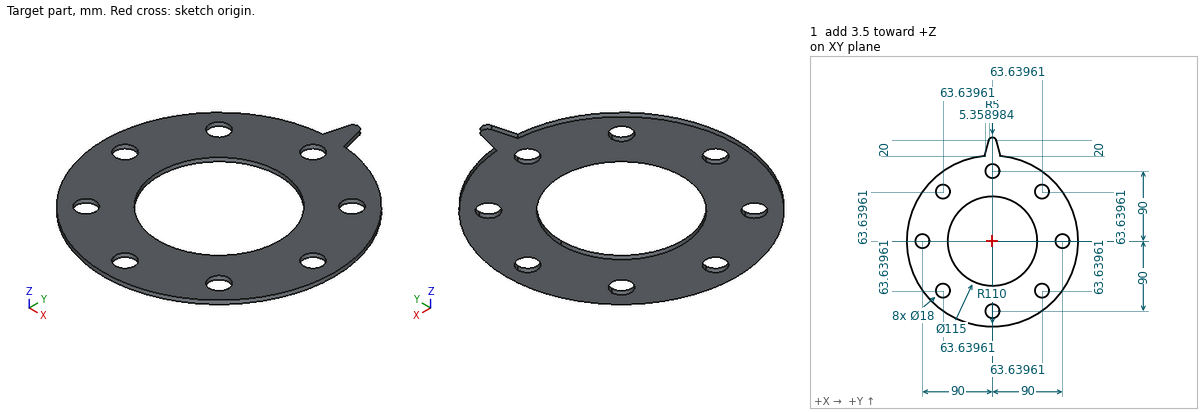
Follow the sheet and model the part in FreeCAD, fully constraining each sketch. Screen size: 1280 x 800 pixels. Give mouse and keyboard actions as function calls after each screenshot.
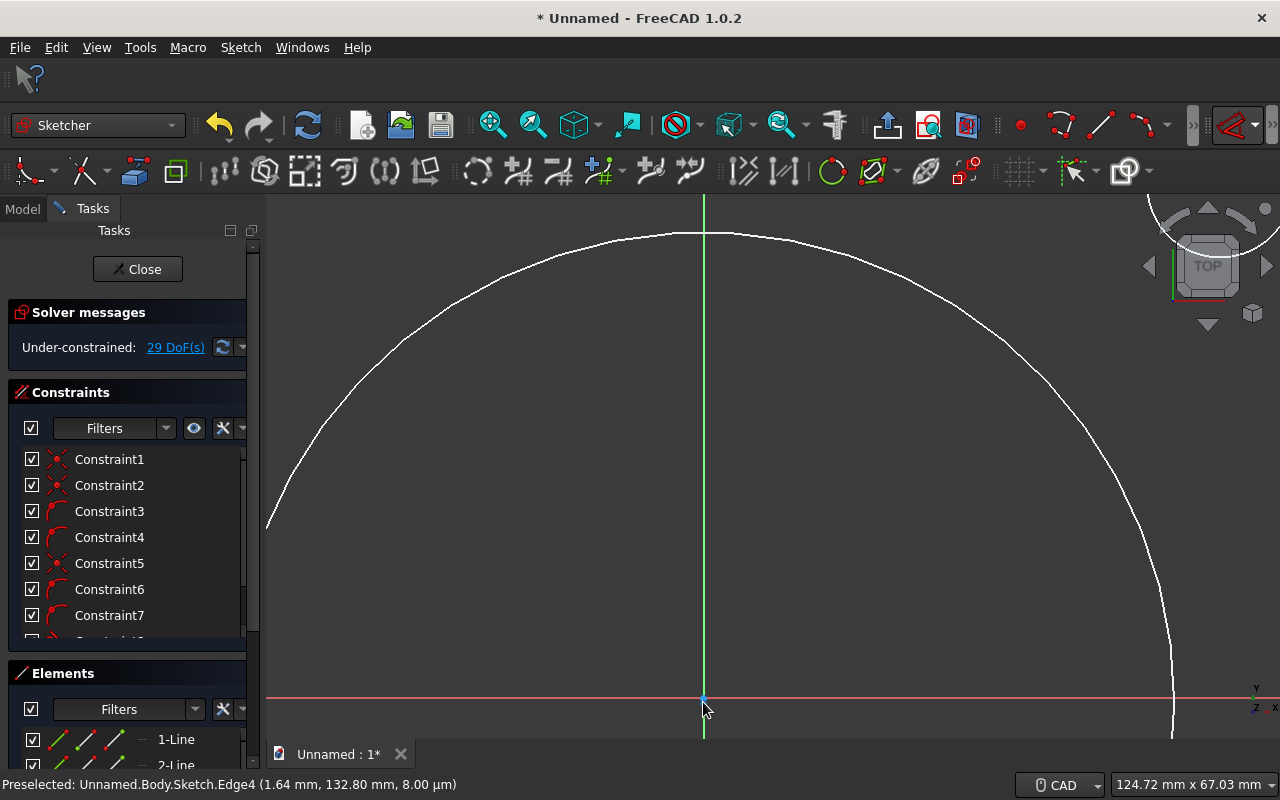
drag(693, 688, 714, 713)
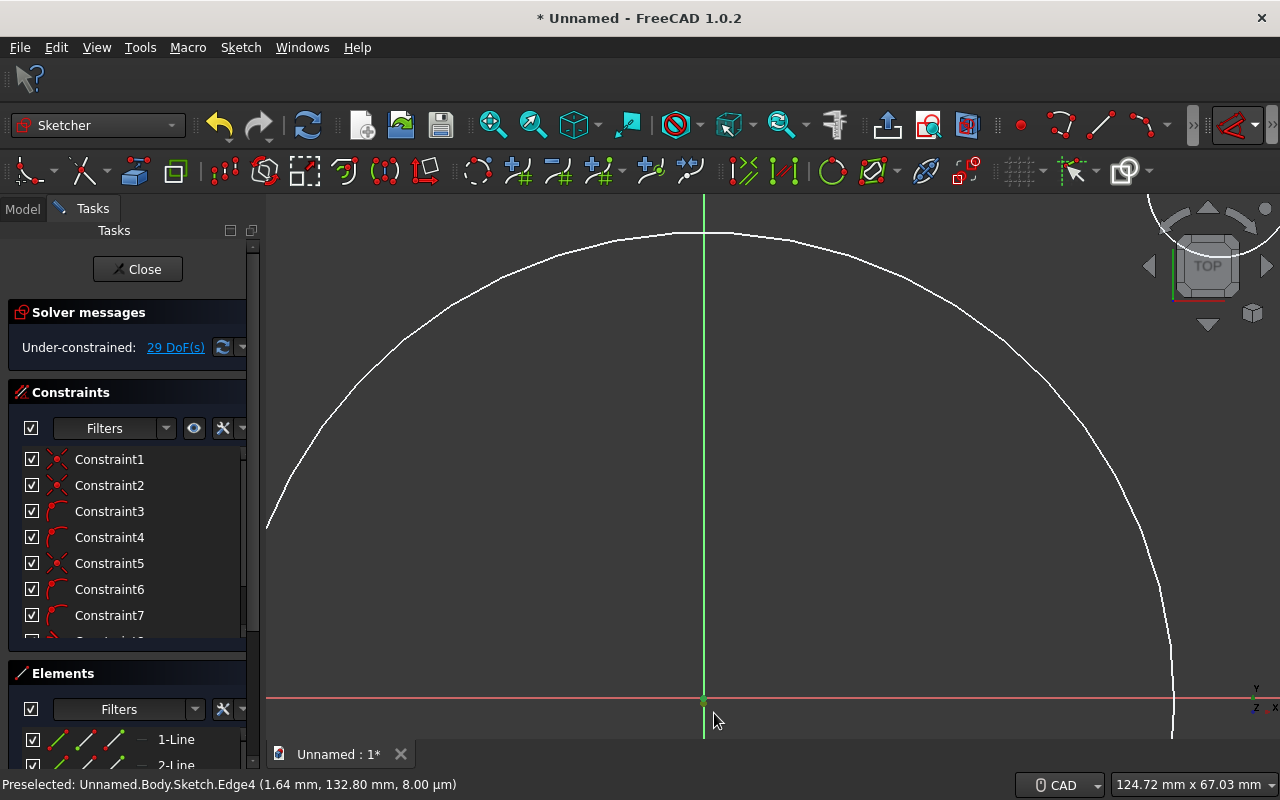
key(c)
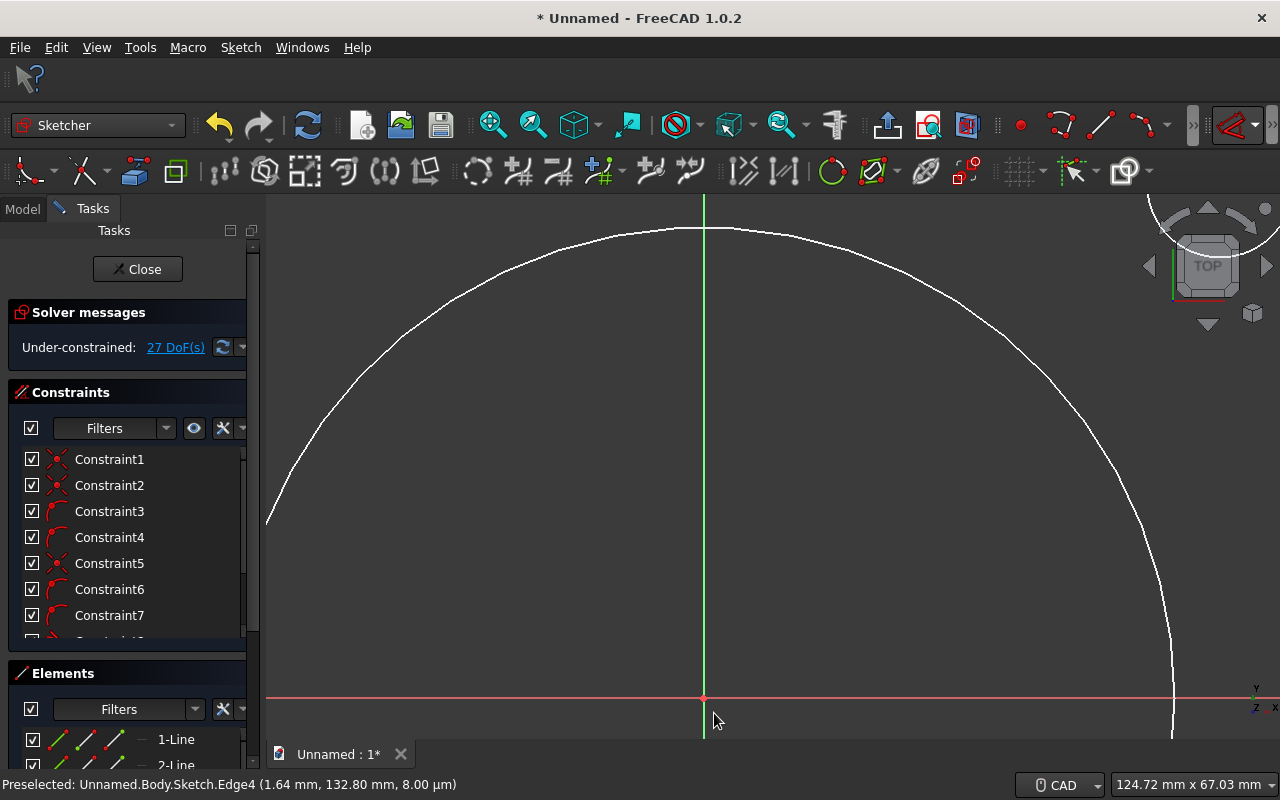
scroll(705, 439, down, 9)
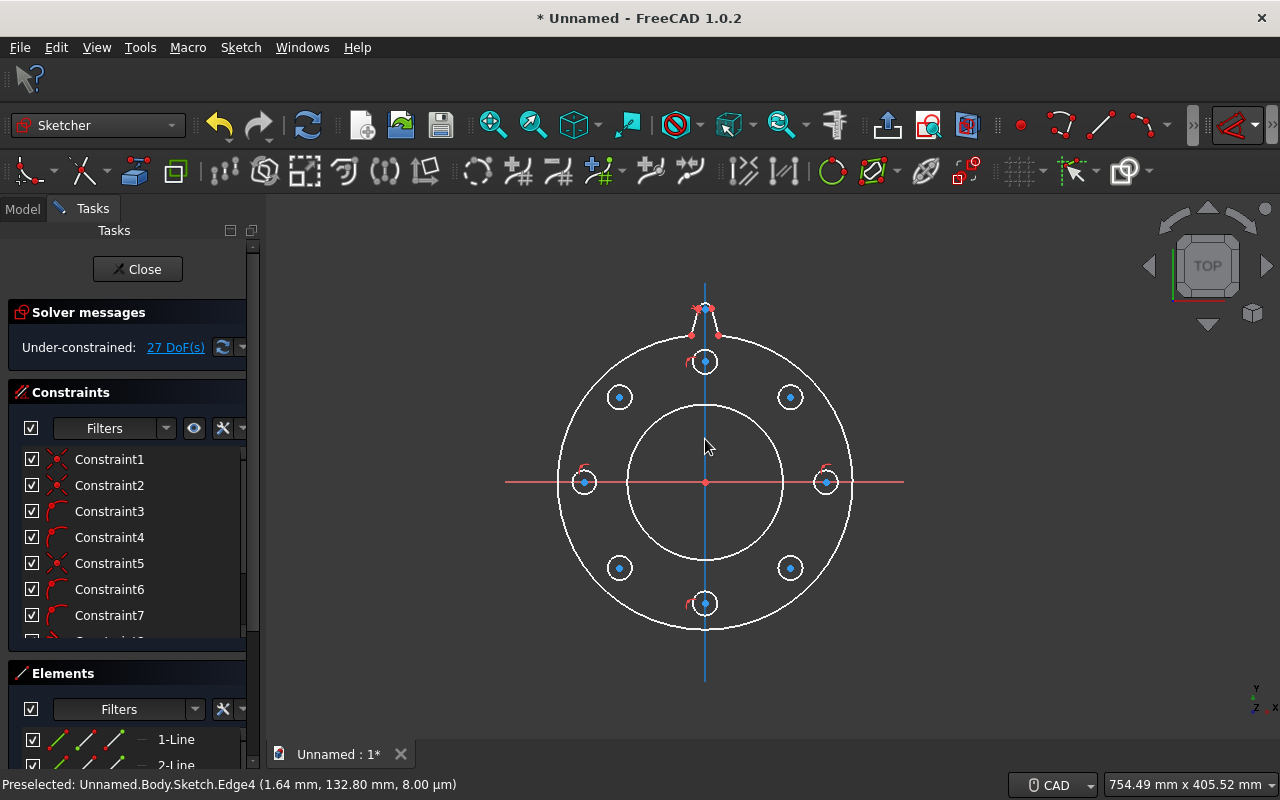
click(628, 559)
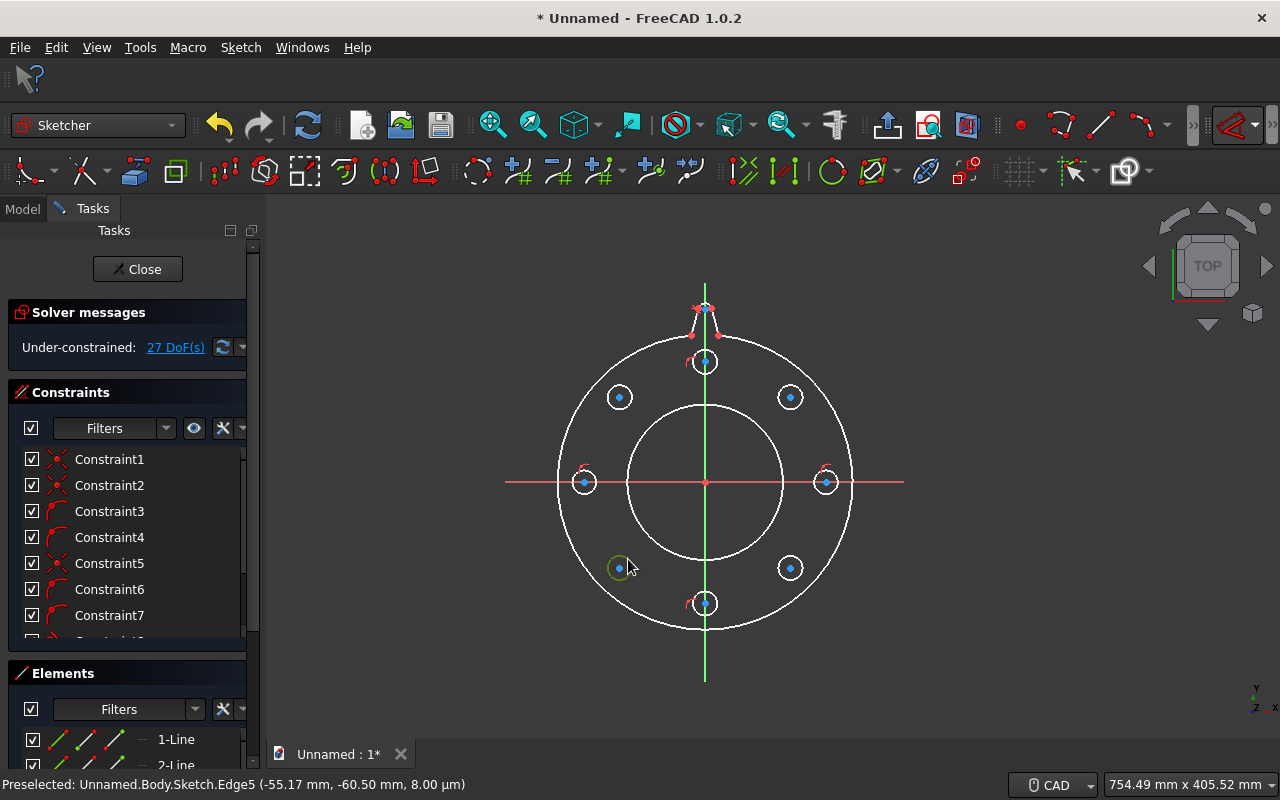
click(705, 591)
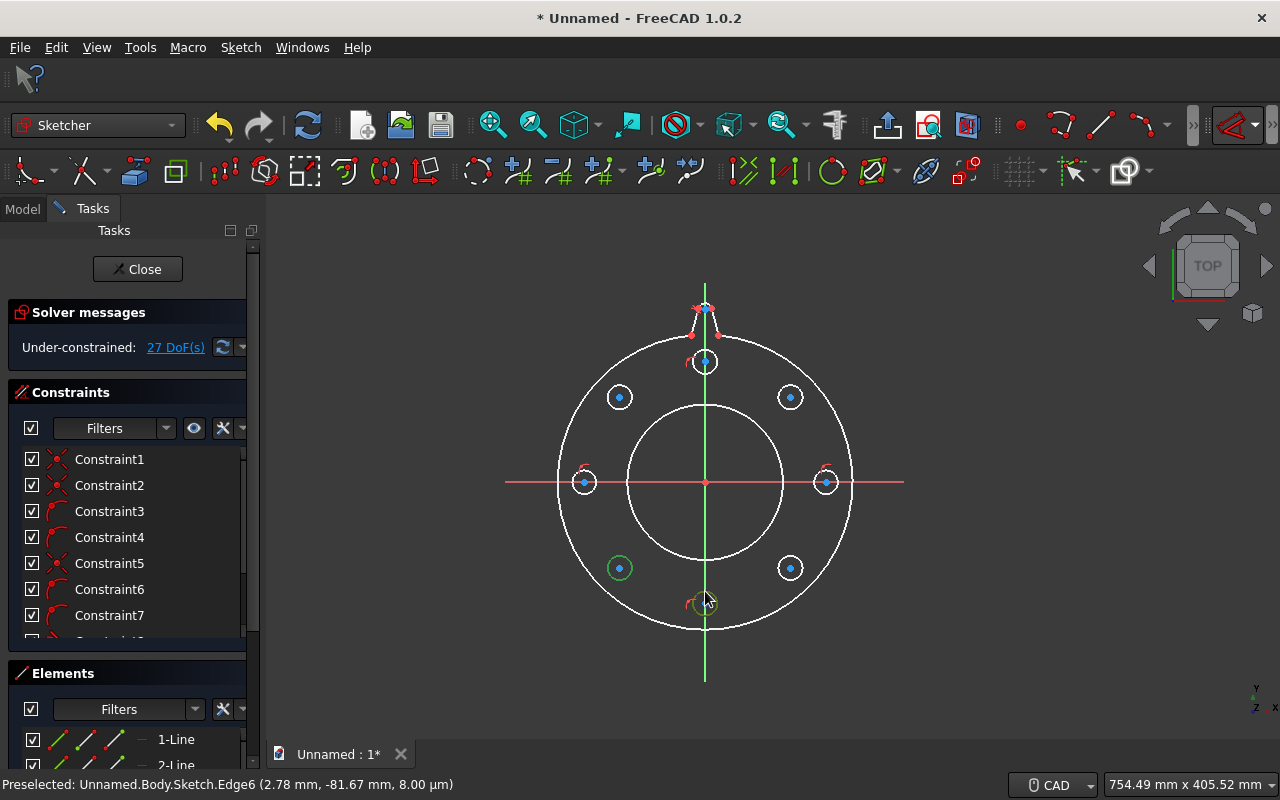
click(799, 559)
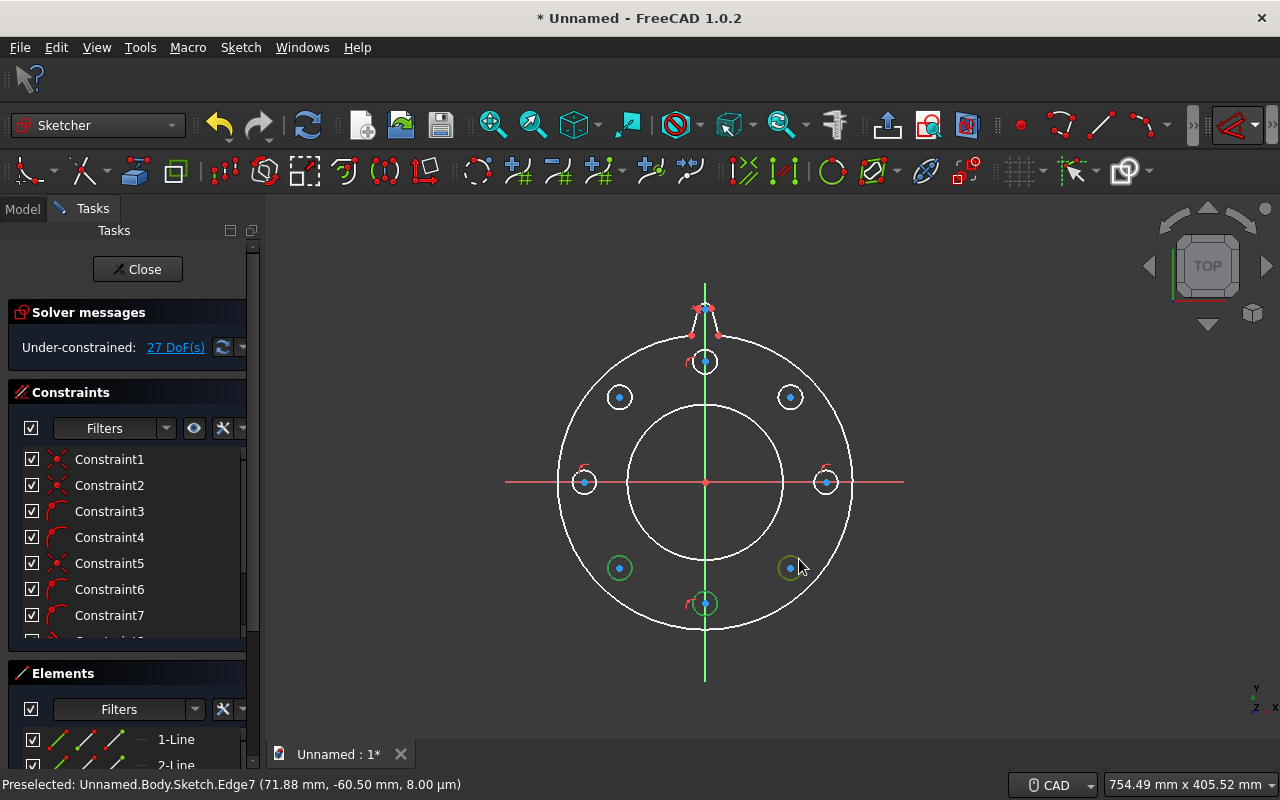
click(572, 482)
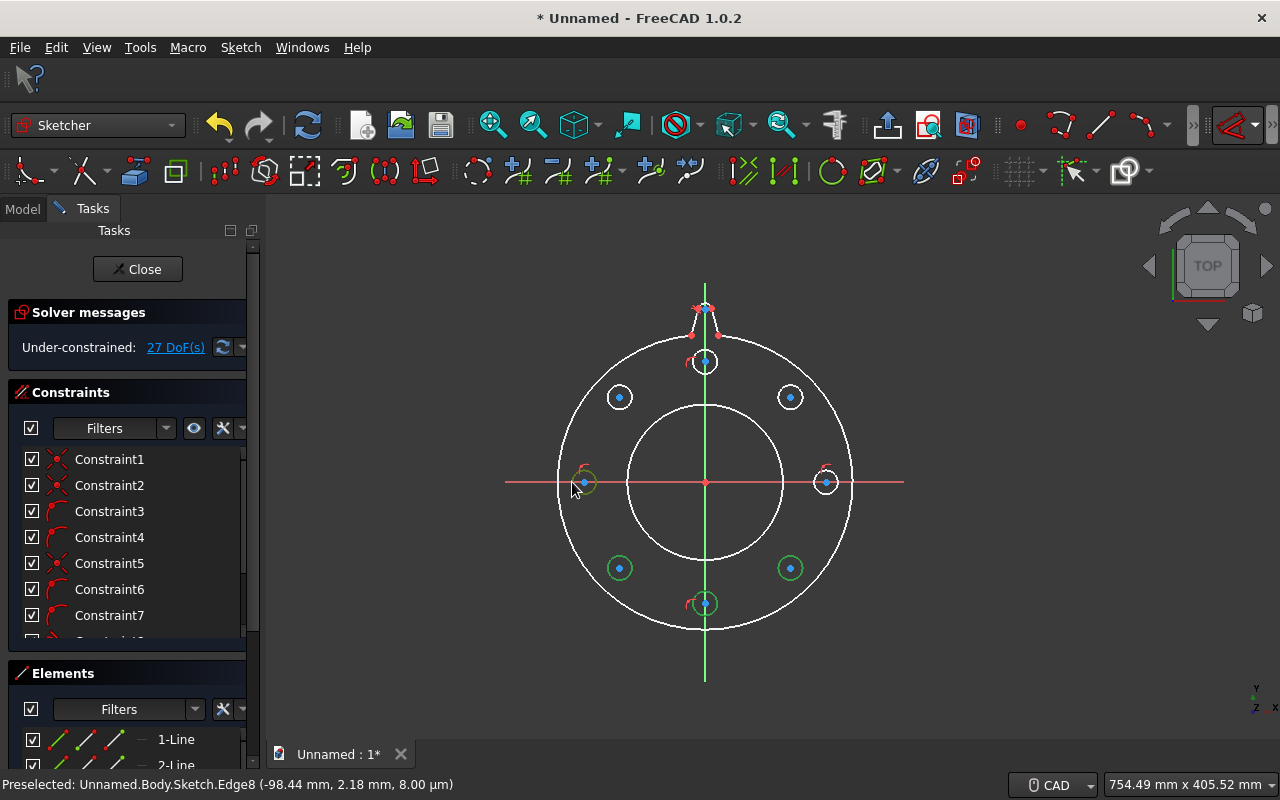
click(628, 389)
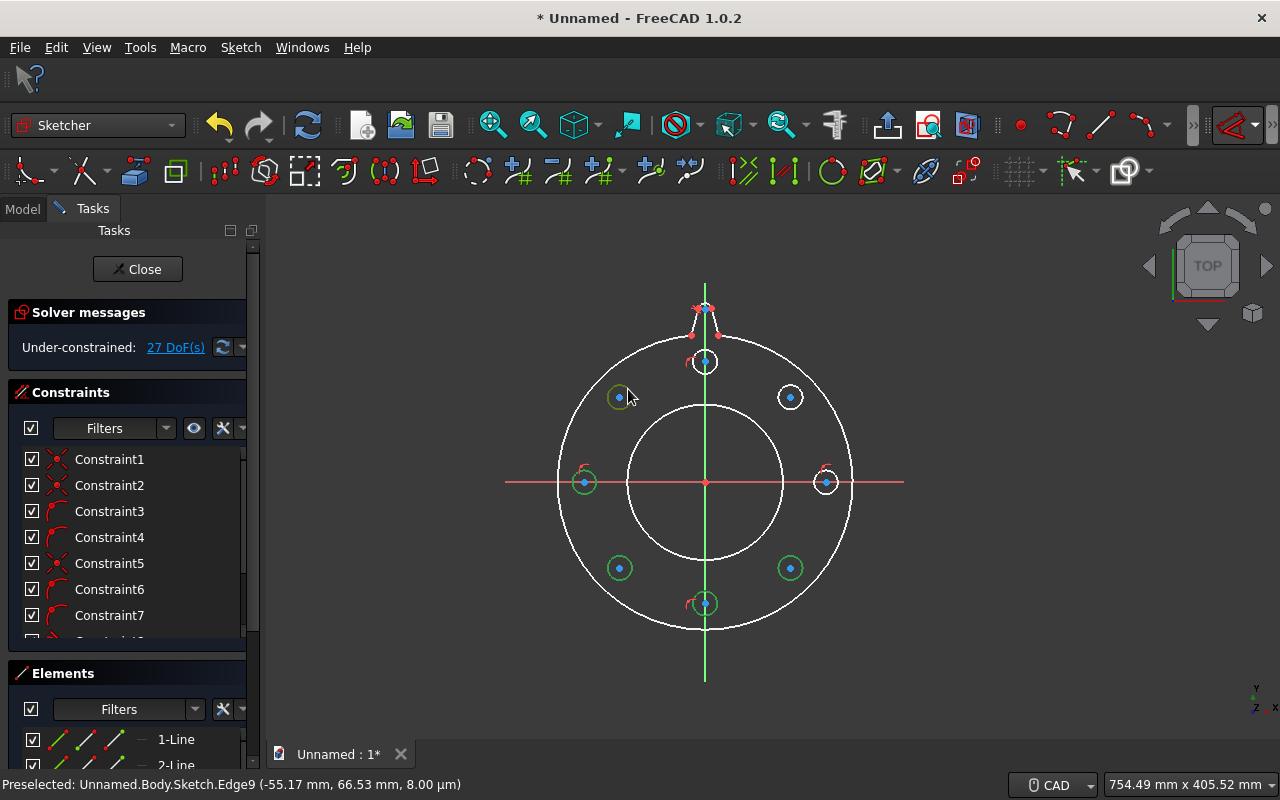
click(814, 482)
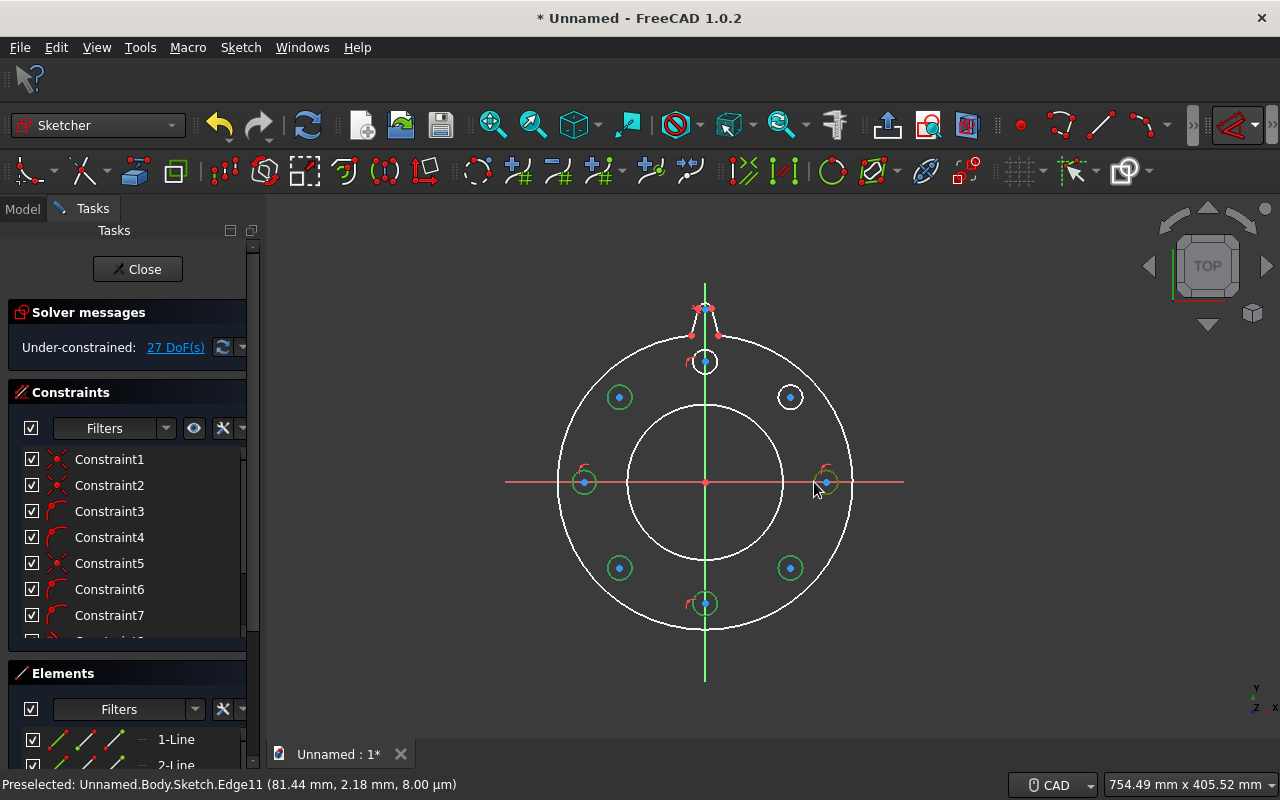
click(705, 350)